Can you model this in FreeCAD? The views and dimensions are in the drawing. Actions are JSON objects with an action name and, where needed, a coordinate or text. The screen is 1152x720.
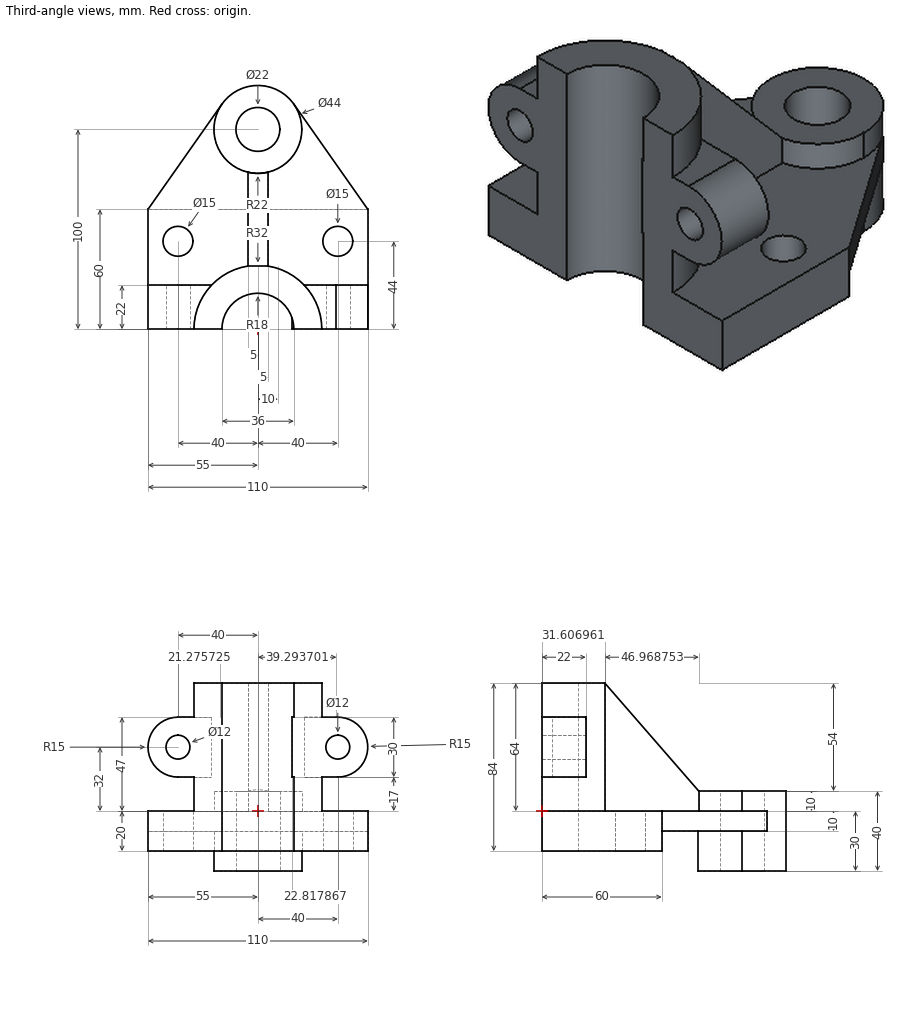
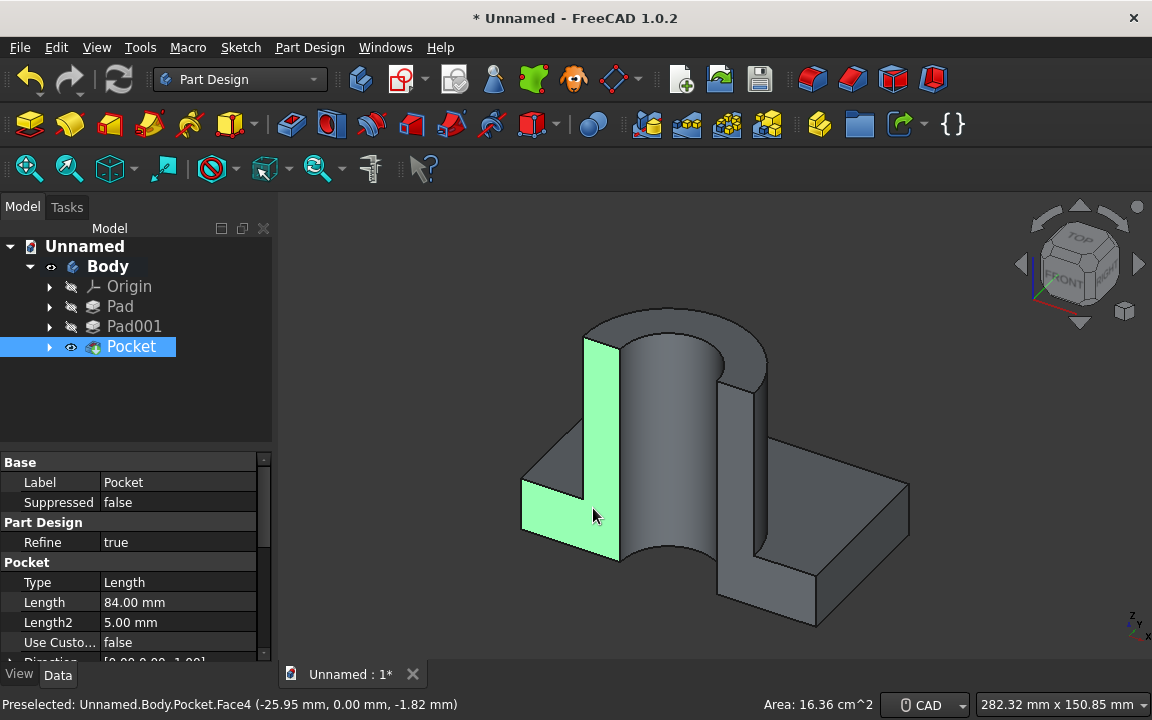
{"action": "left_click", "coordinate": [402, 80]}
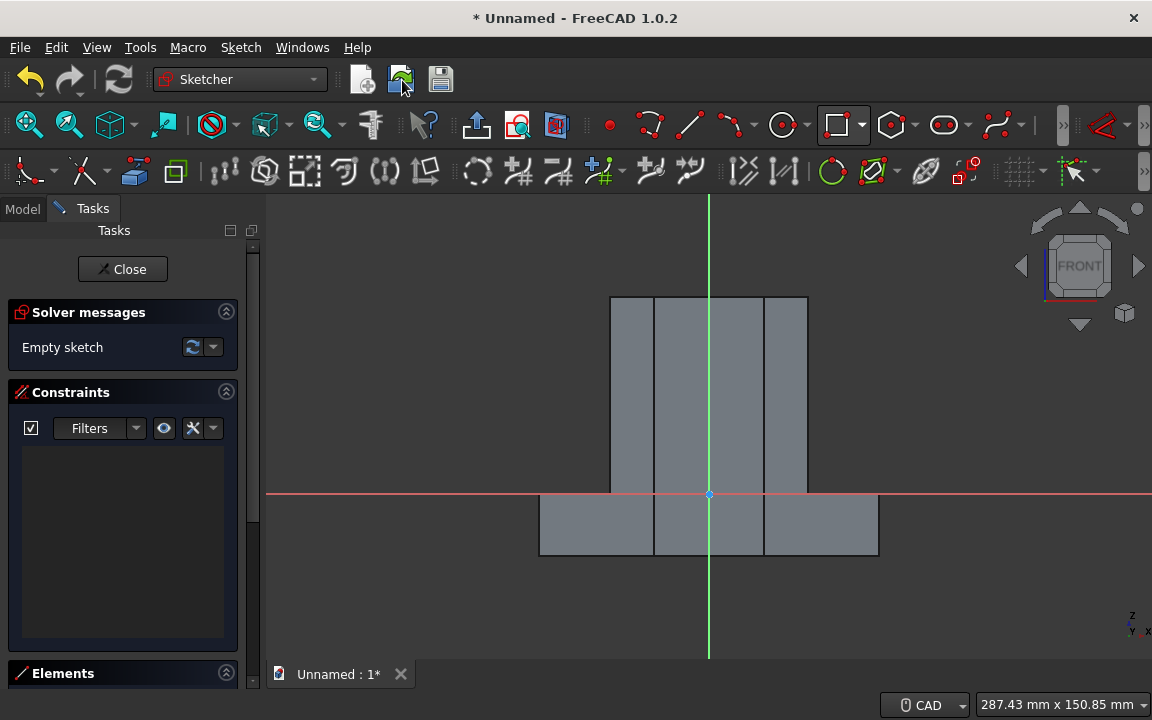
{"action": "scroll", "coordinate": [604, 416], "scroll_direction": "up", "scroll_amount": 3}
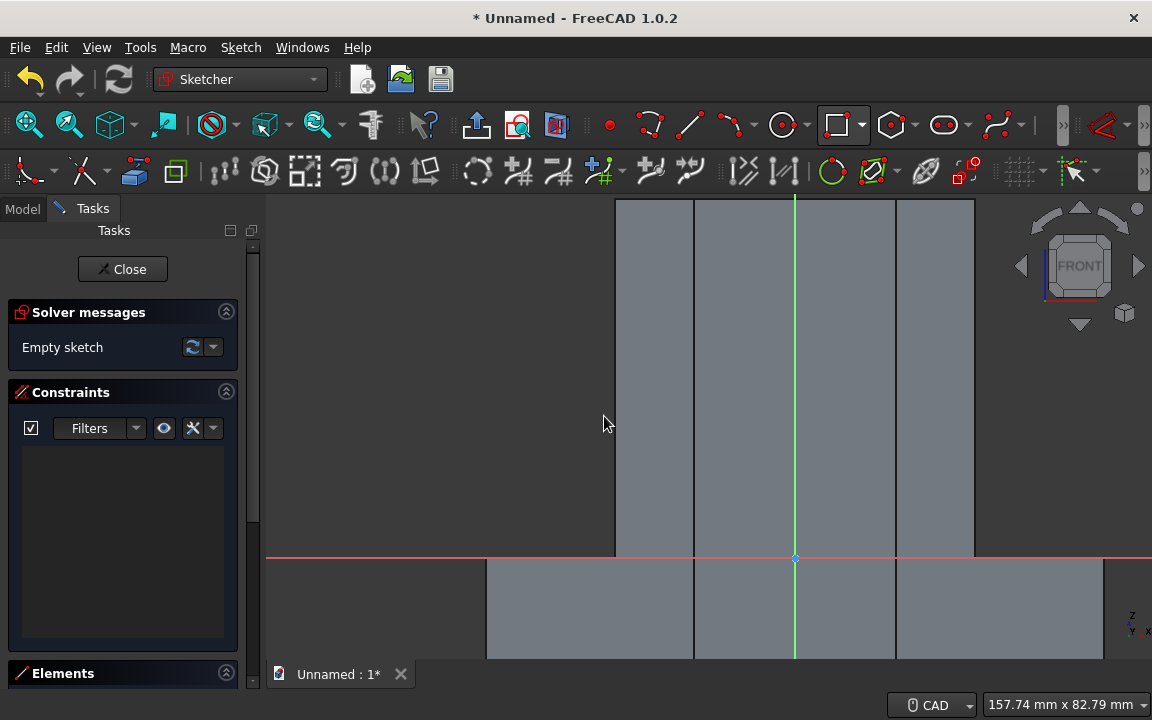
{"action": "left_click", "coordinate": [650, 126]}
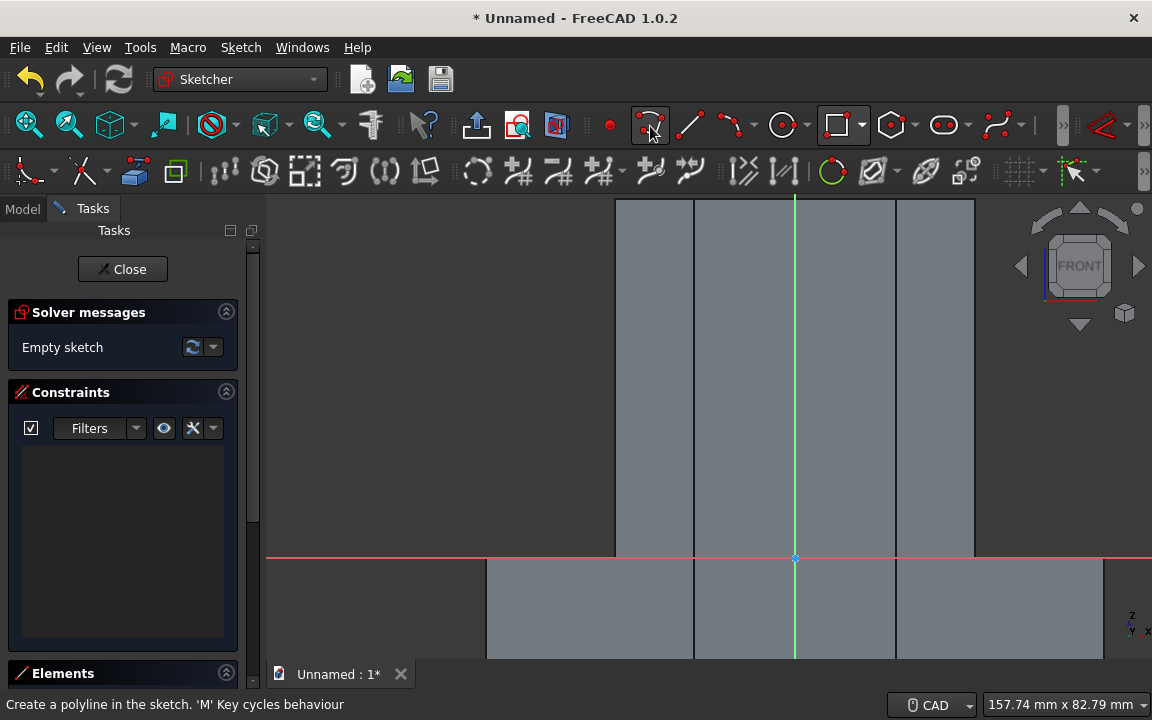
{"action": "left_click", "coordinate": [570, 294]}
{"action": "left_click", "coordinate": [690, 294]}
{"action": "left_click", "coordinate": [690, 463]}
{"action": "left_click", "coordinate": [570, 463]}
{"action": "right_click", "coordinate": [570, 463]}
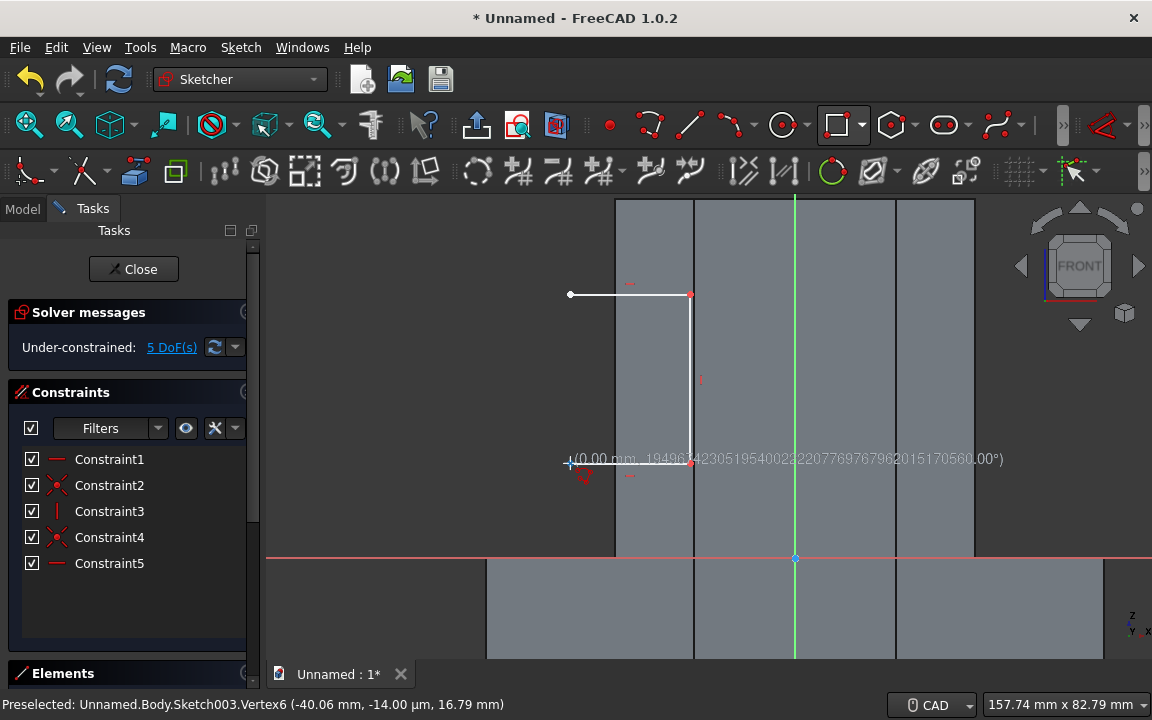
{"action": "left_click", "coordinate": [730, 126]}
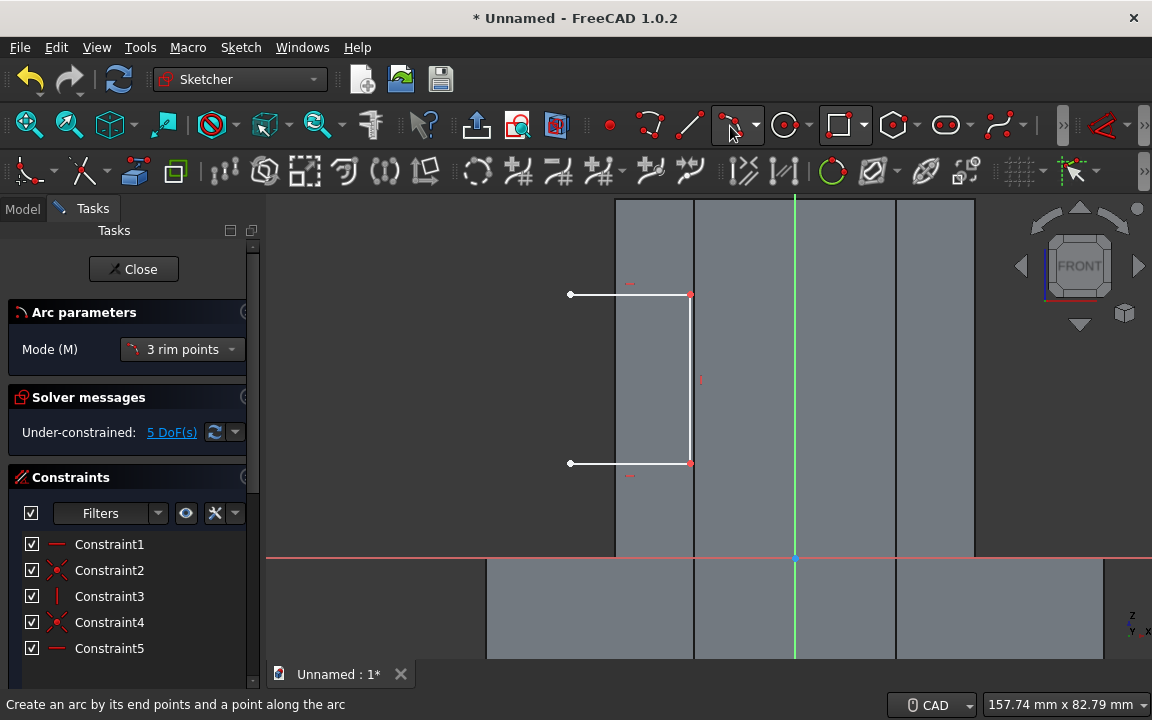
{"action": "left_click", "coordinate": [570, 464]}
{"action": "left_click", "coordinate": [570, 295]}
{"action": "left_click", "coordinate": [486, 379]}
{"action": "key", "text": "Escape"}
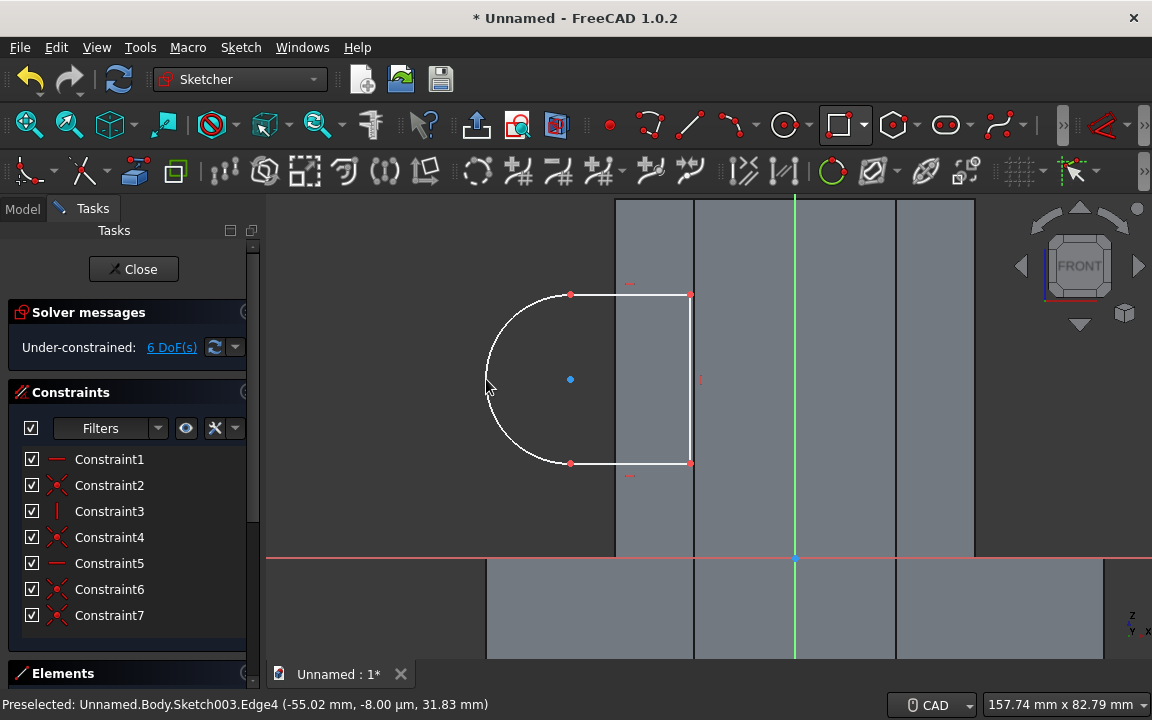
{"action": "left_click", "coordinate": [606, 295]}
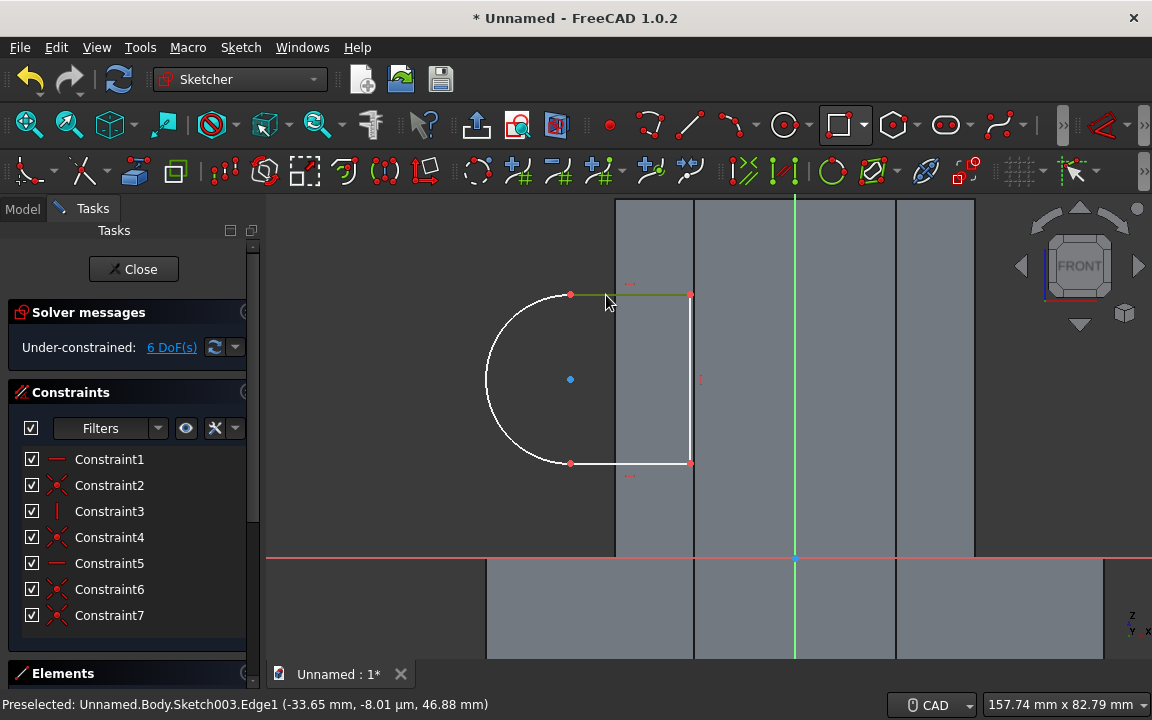
{"action": "left_click", "coordinate": [502, 330]}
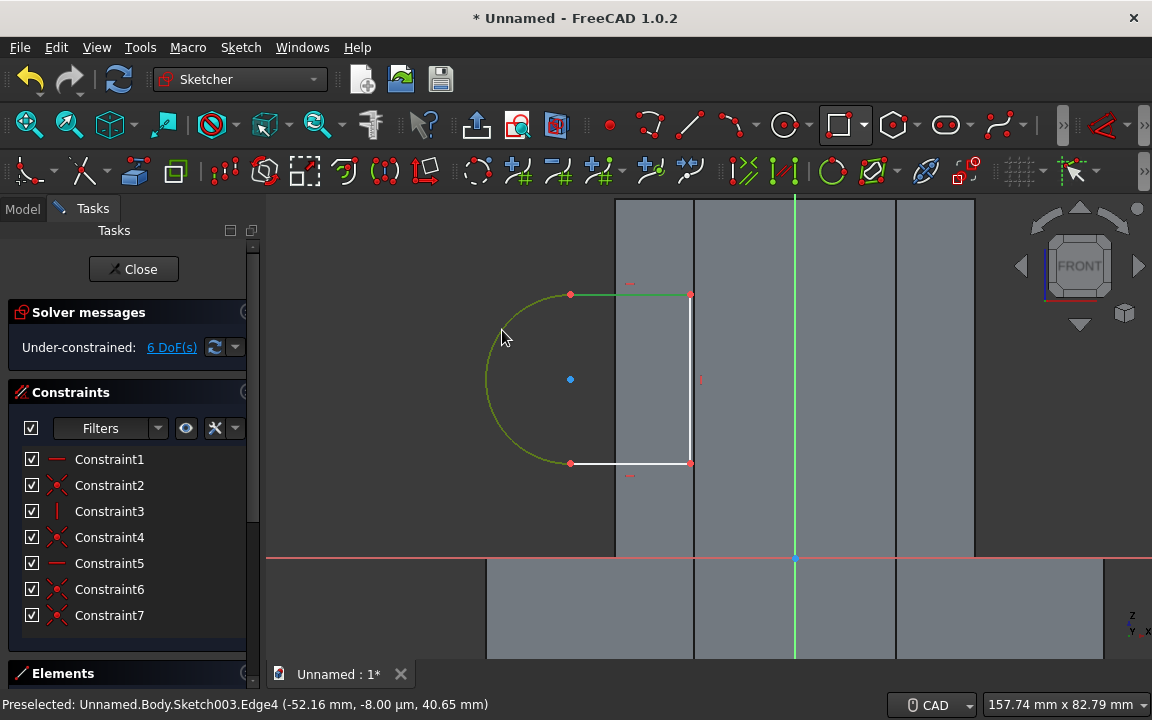
{"action": "key", "text": "t"}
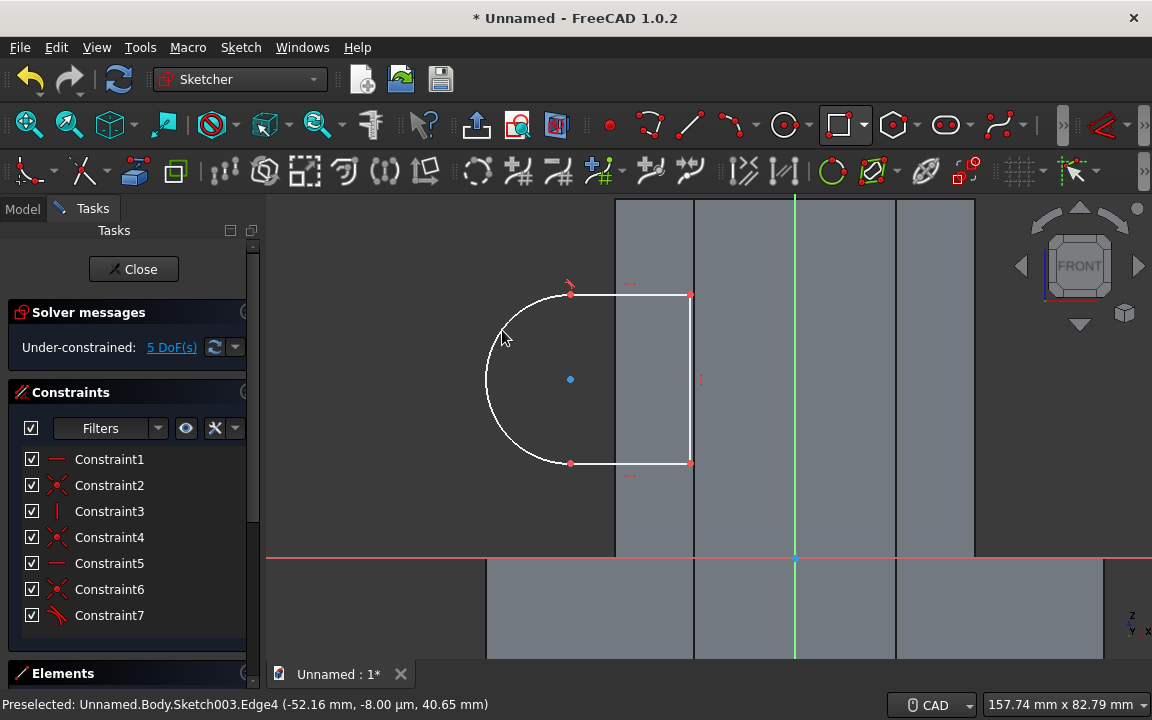
{"action": "left_click", "coordinate": [654, 464]}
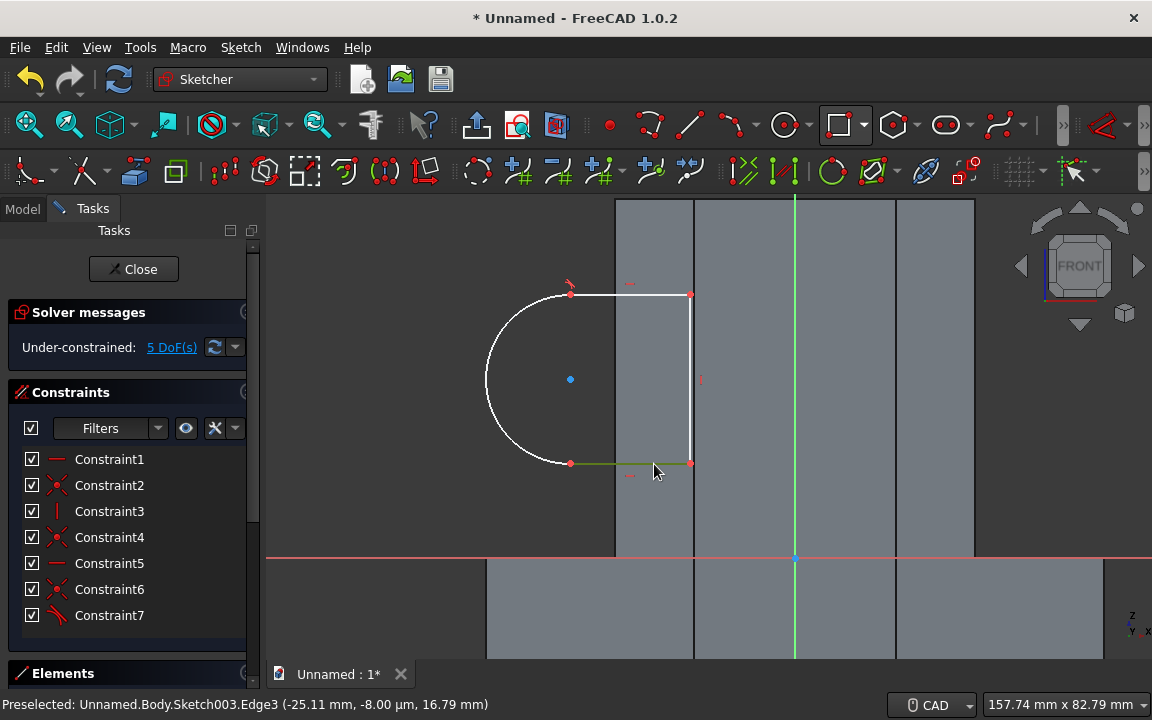
{"action": "left_click", "coordinate": [502, 330]}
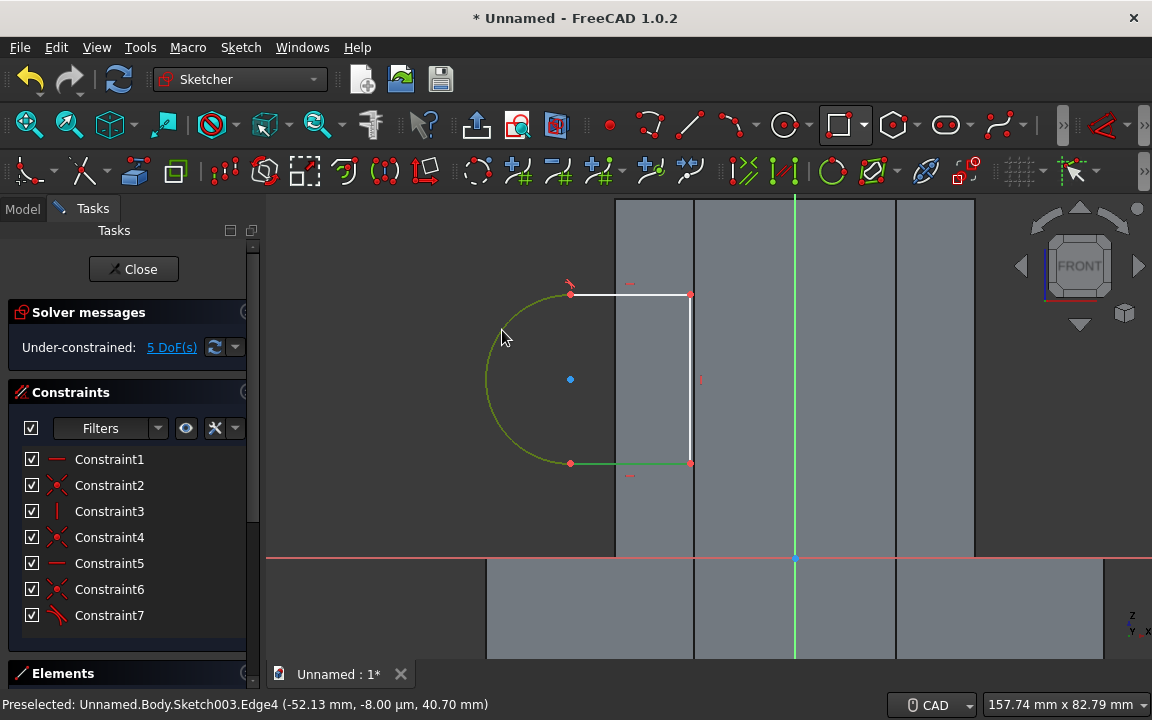
{"action": "key", "text": "t"}